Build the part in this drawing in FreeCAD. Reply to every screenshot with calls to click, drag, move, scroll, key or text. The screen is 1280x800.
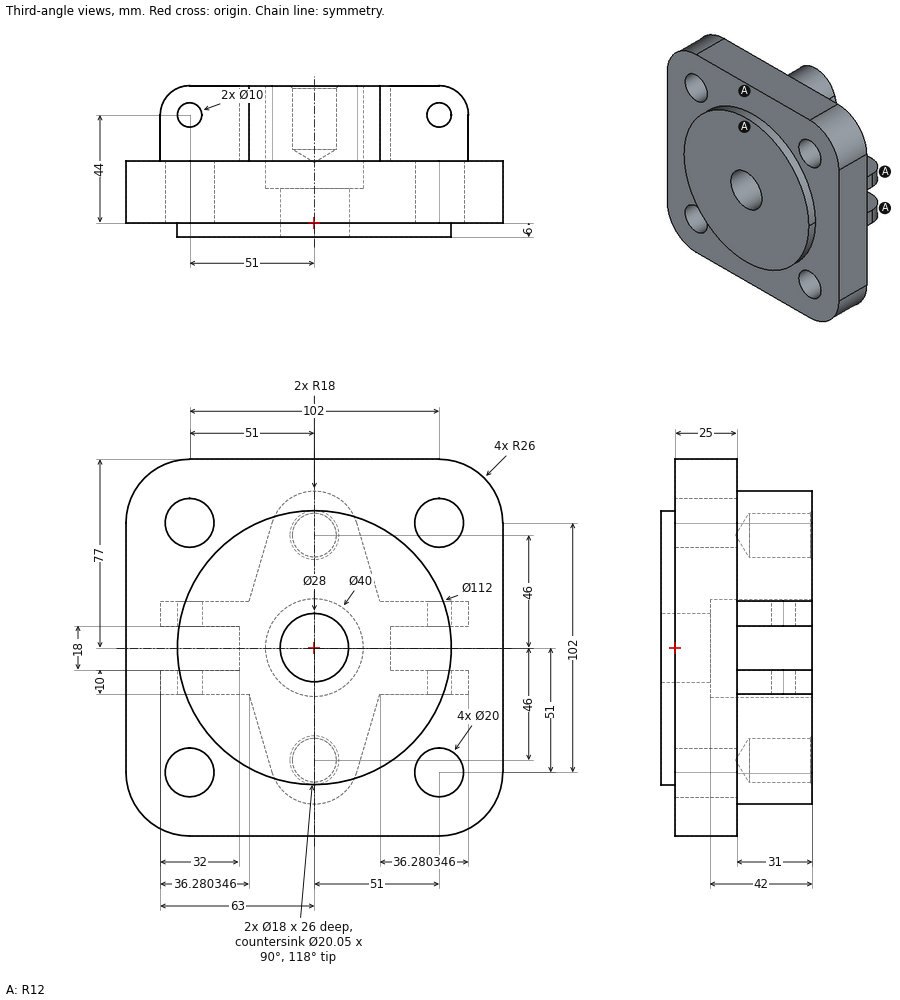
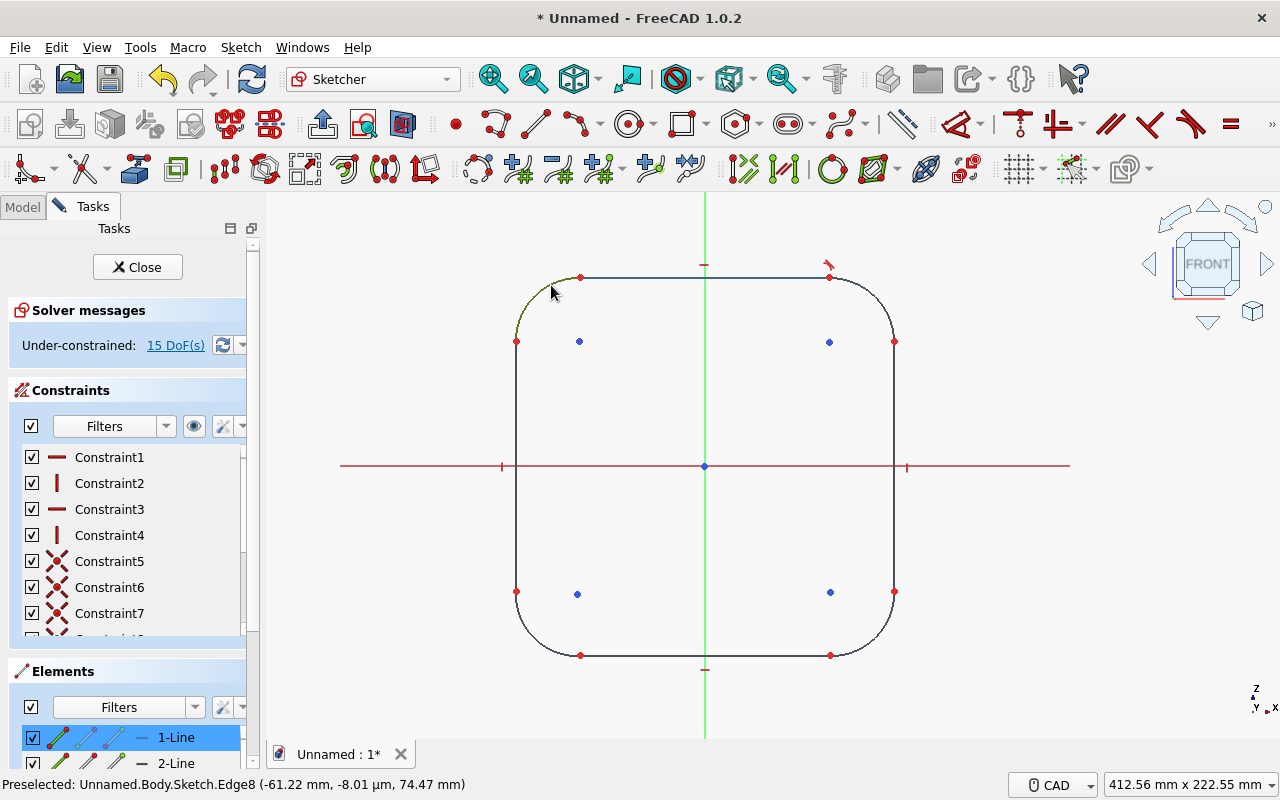
click(1192, 124)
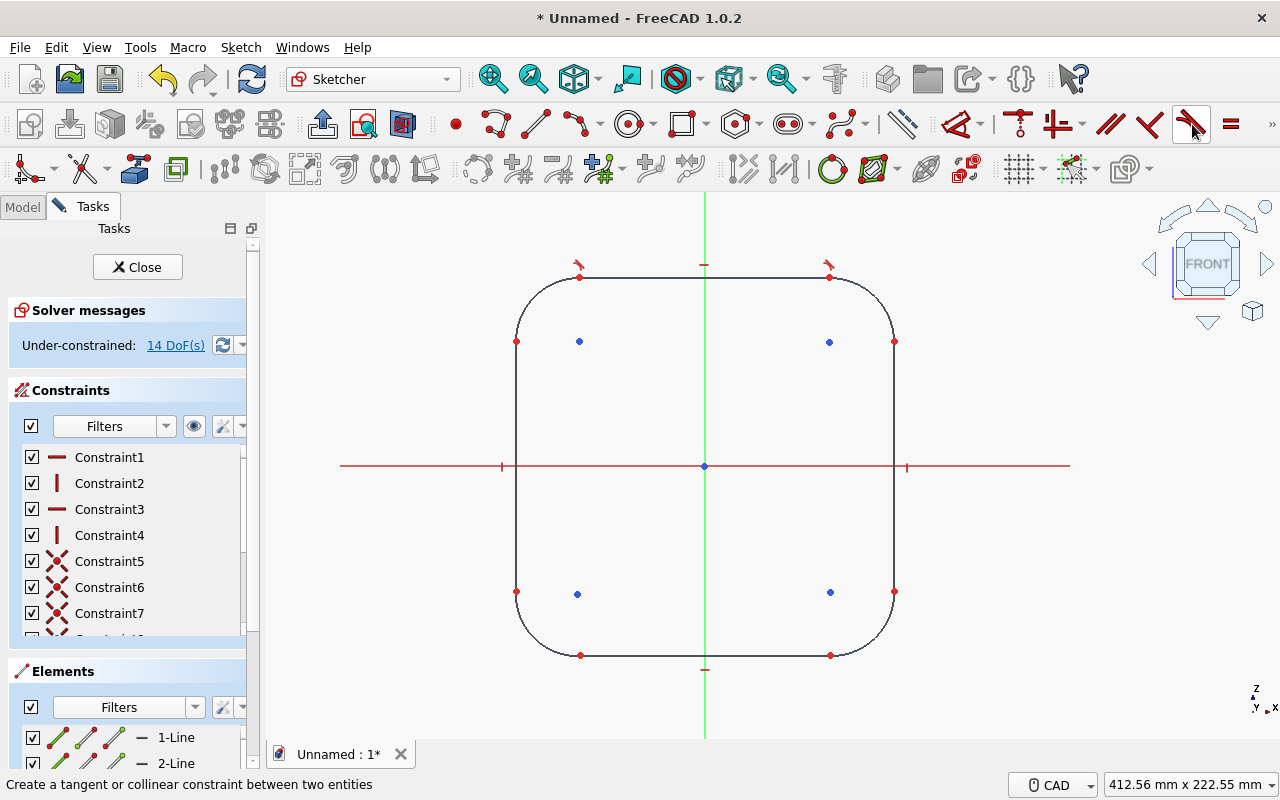
click(894, 417)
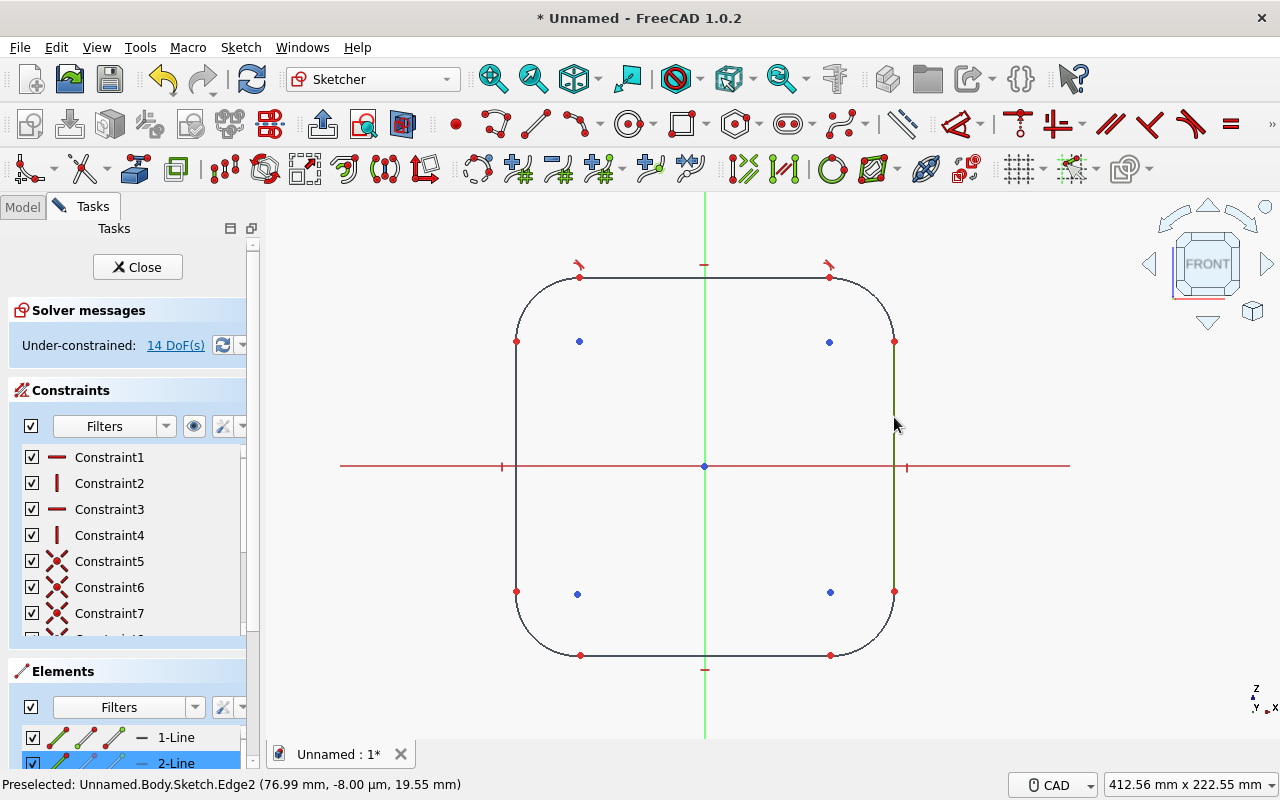
click(887, 313)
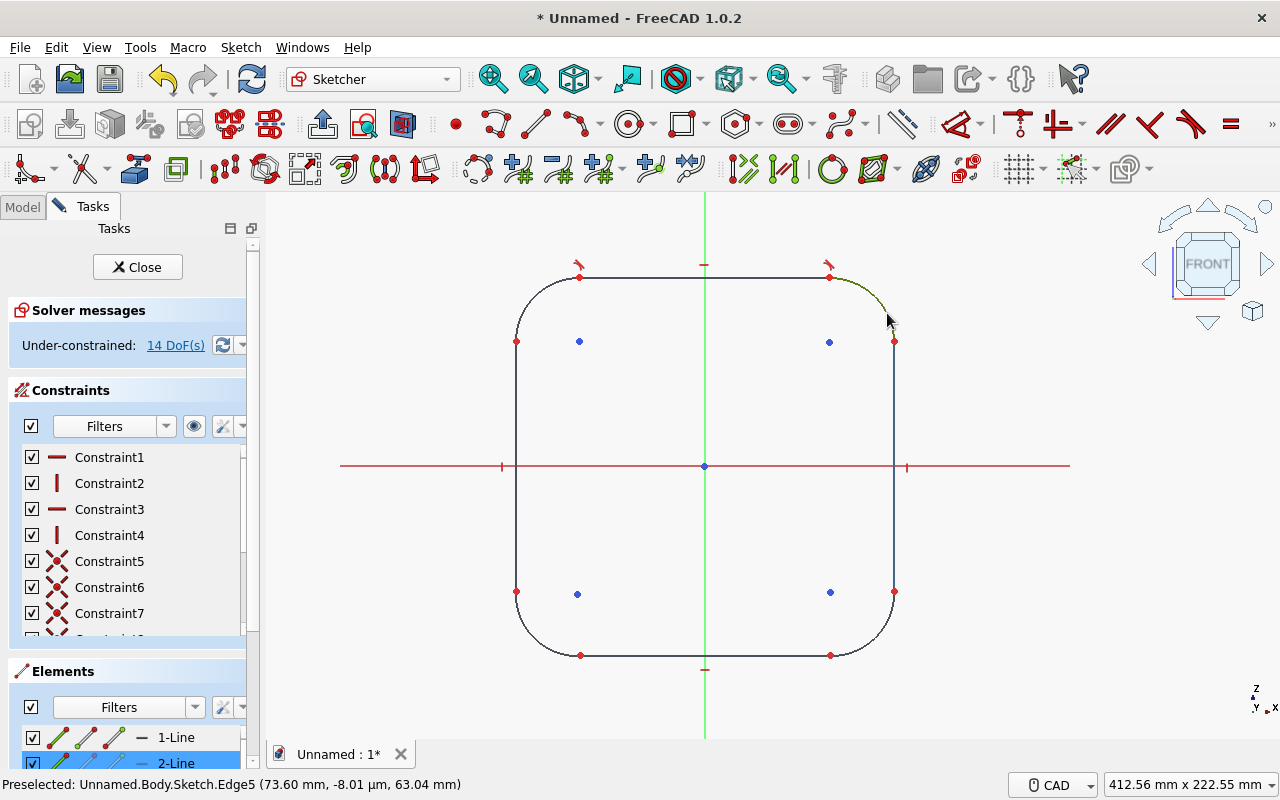
click(1192, 124)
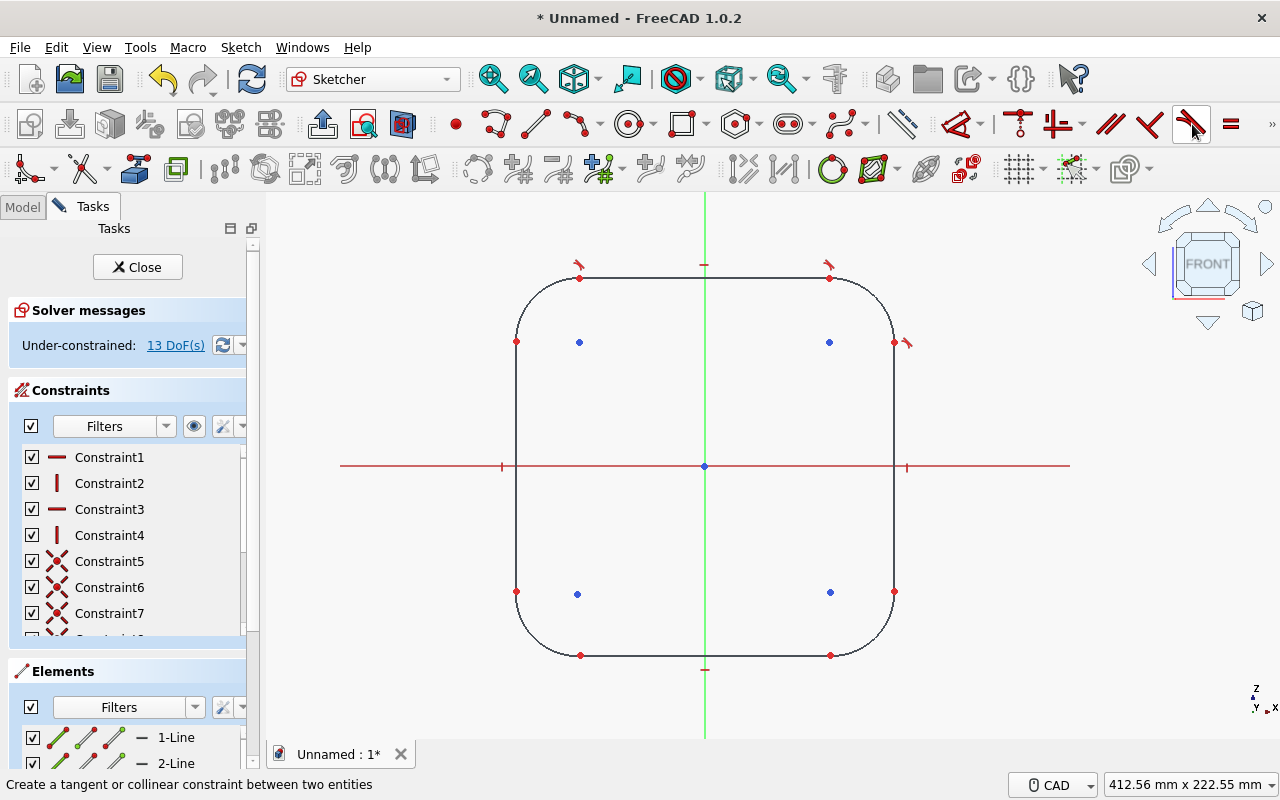
click(894, 418)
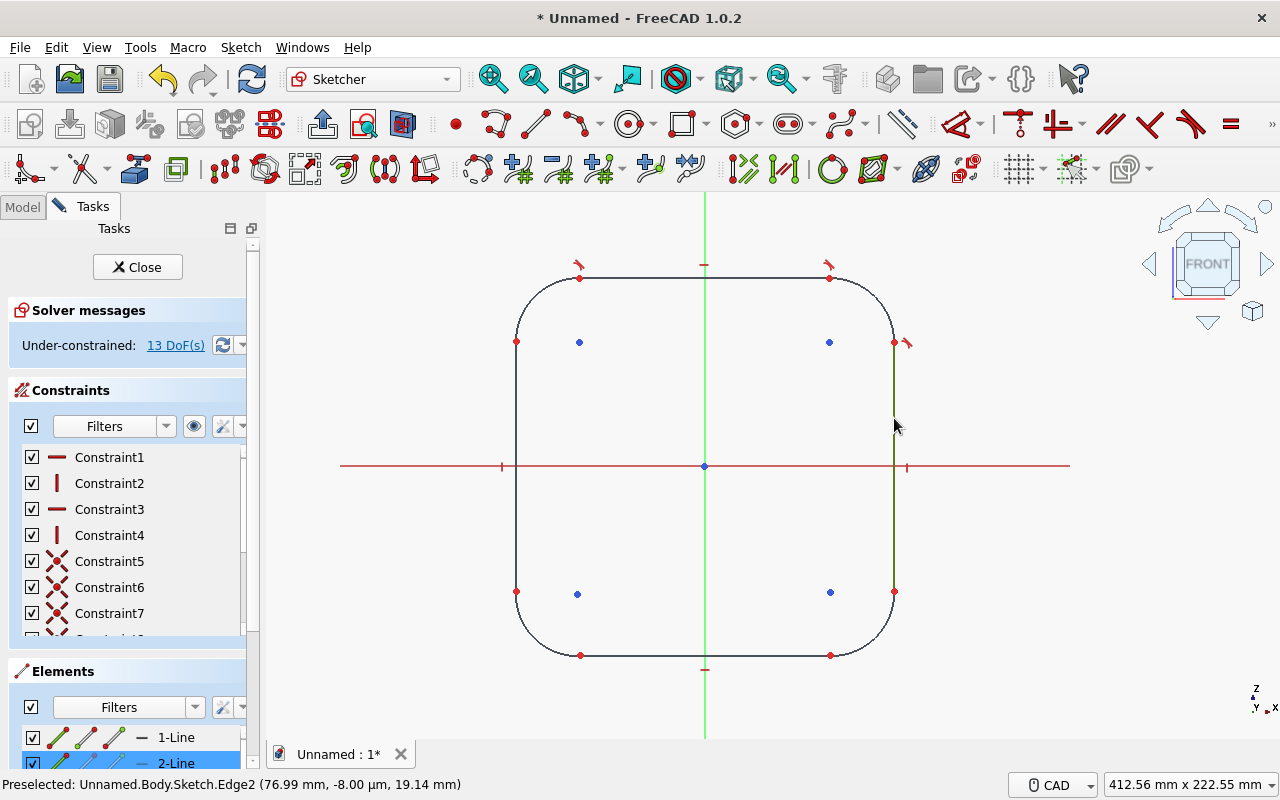
click(859, 649)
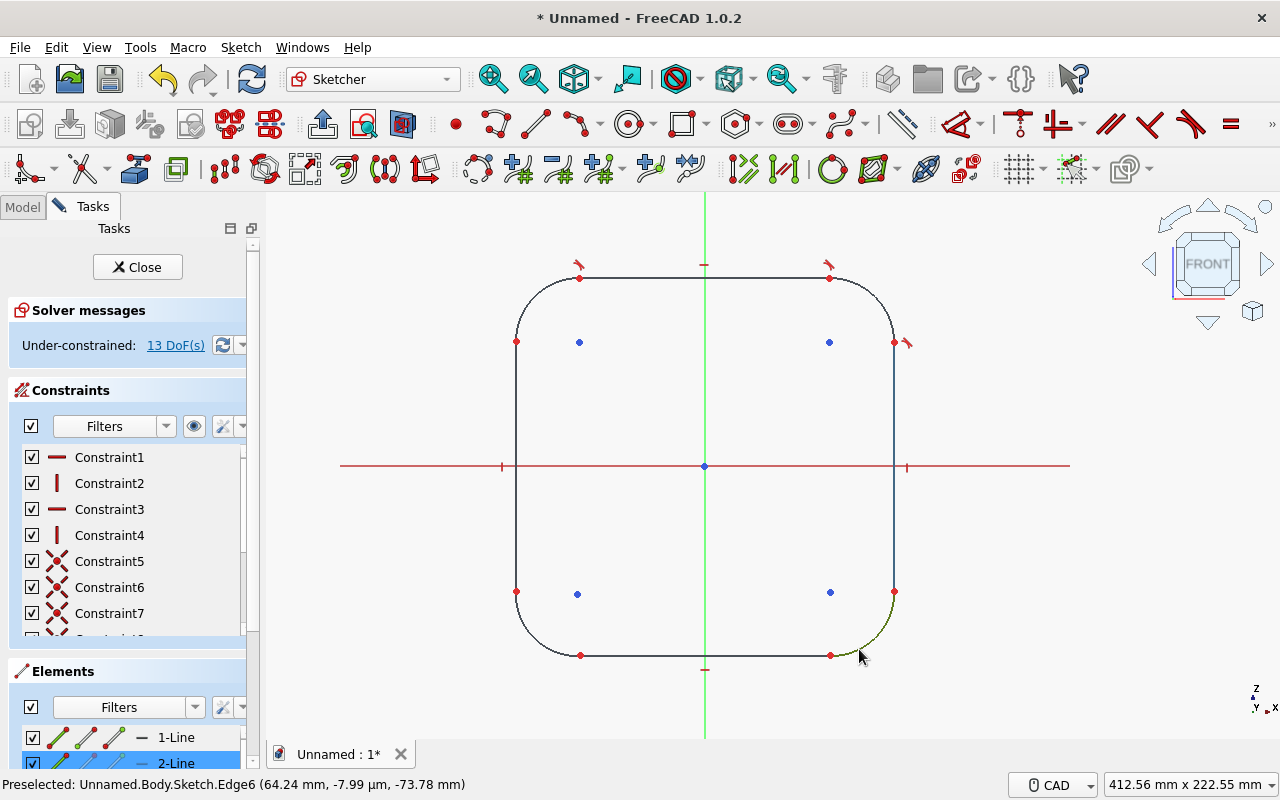
key(t)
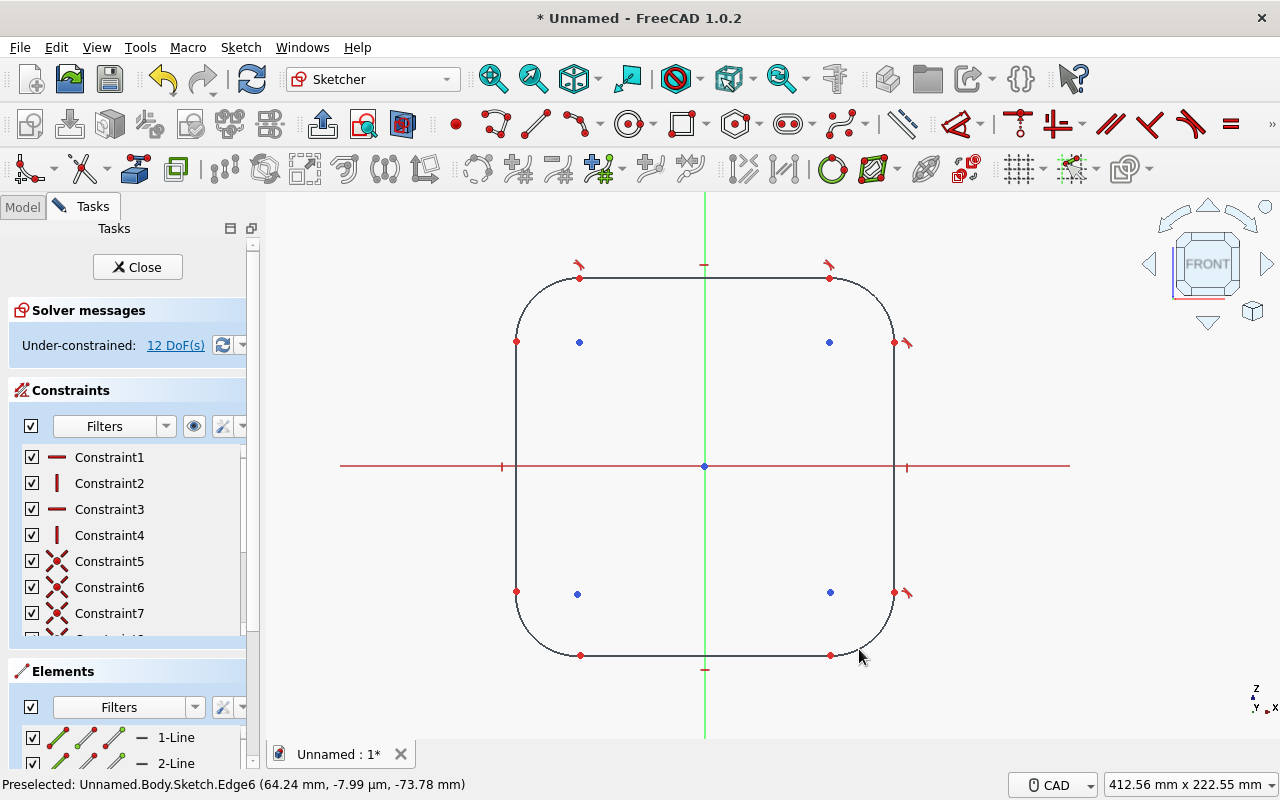
click(755, 656)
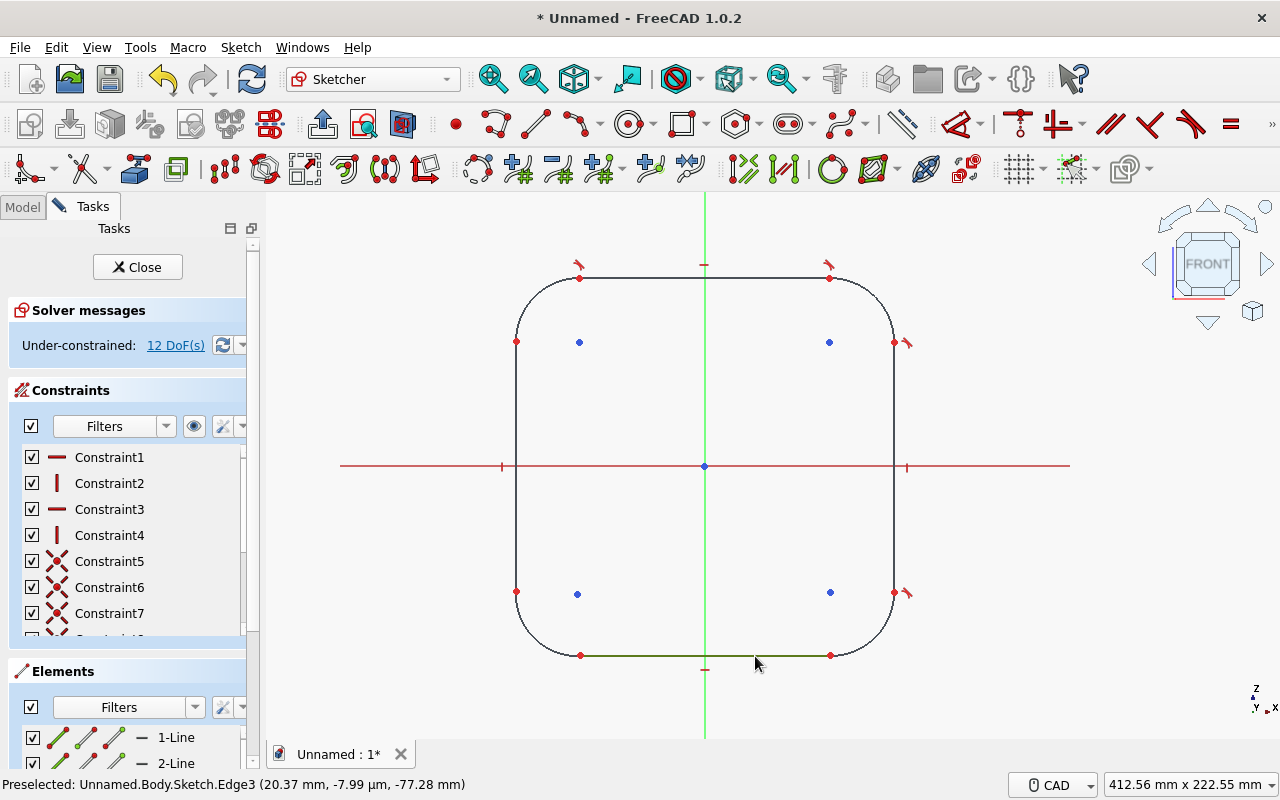
click(859, 649)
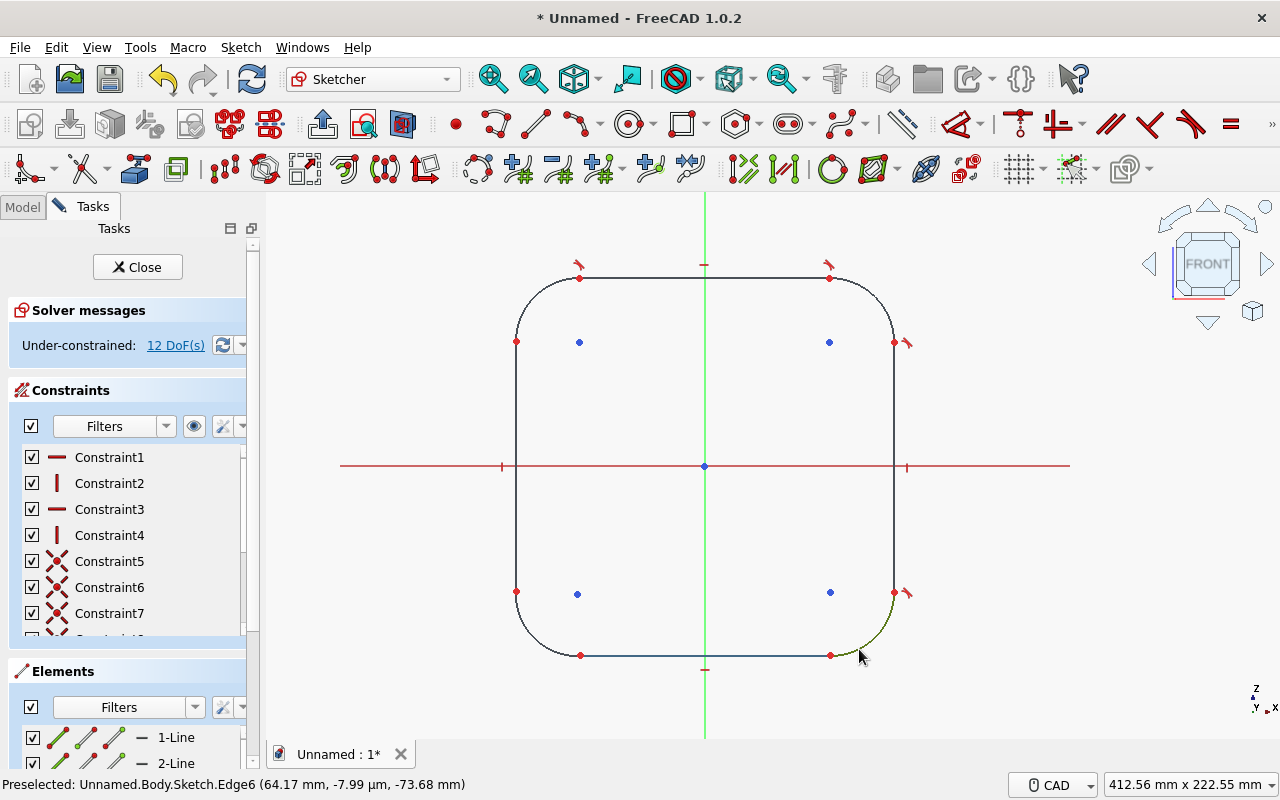
key(t)